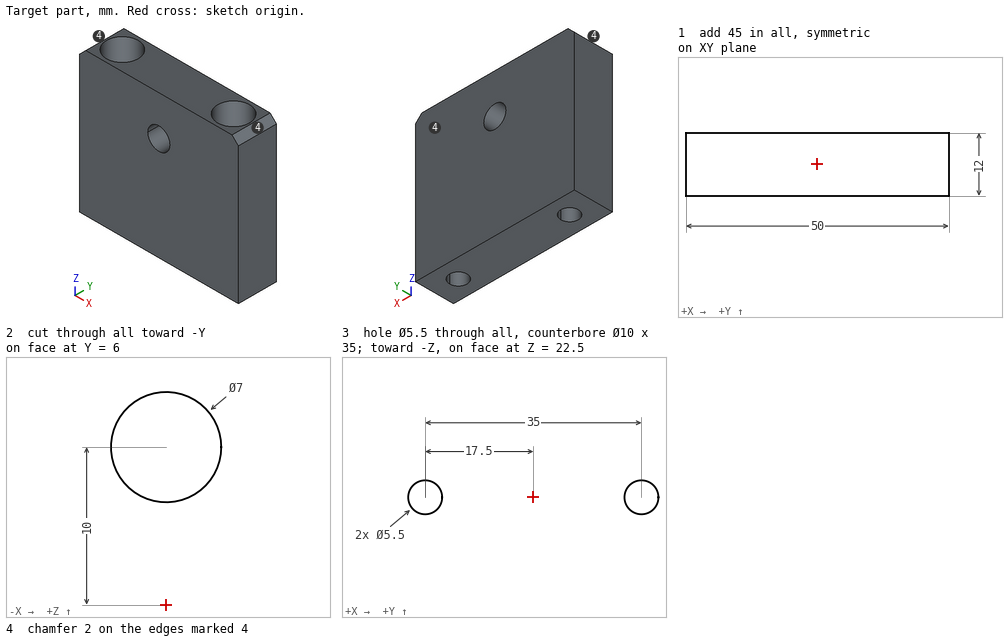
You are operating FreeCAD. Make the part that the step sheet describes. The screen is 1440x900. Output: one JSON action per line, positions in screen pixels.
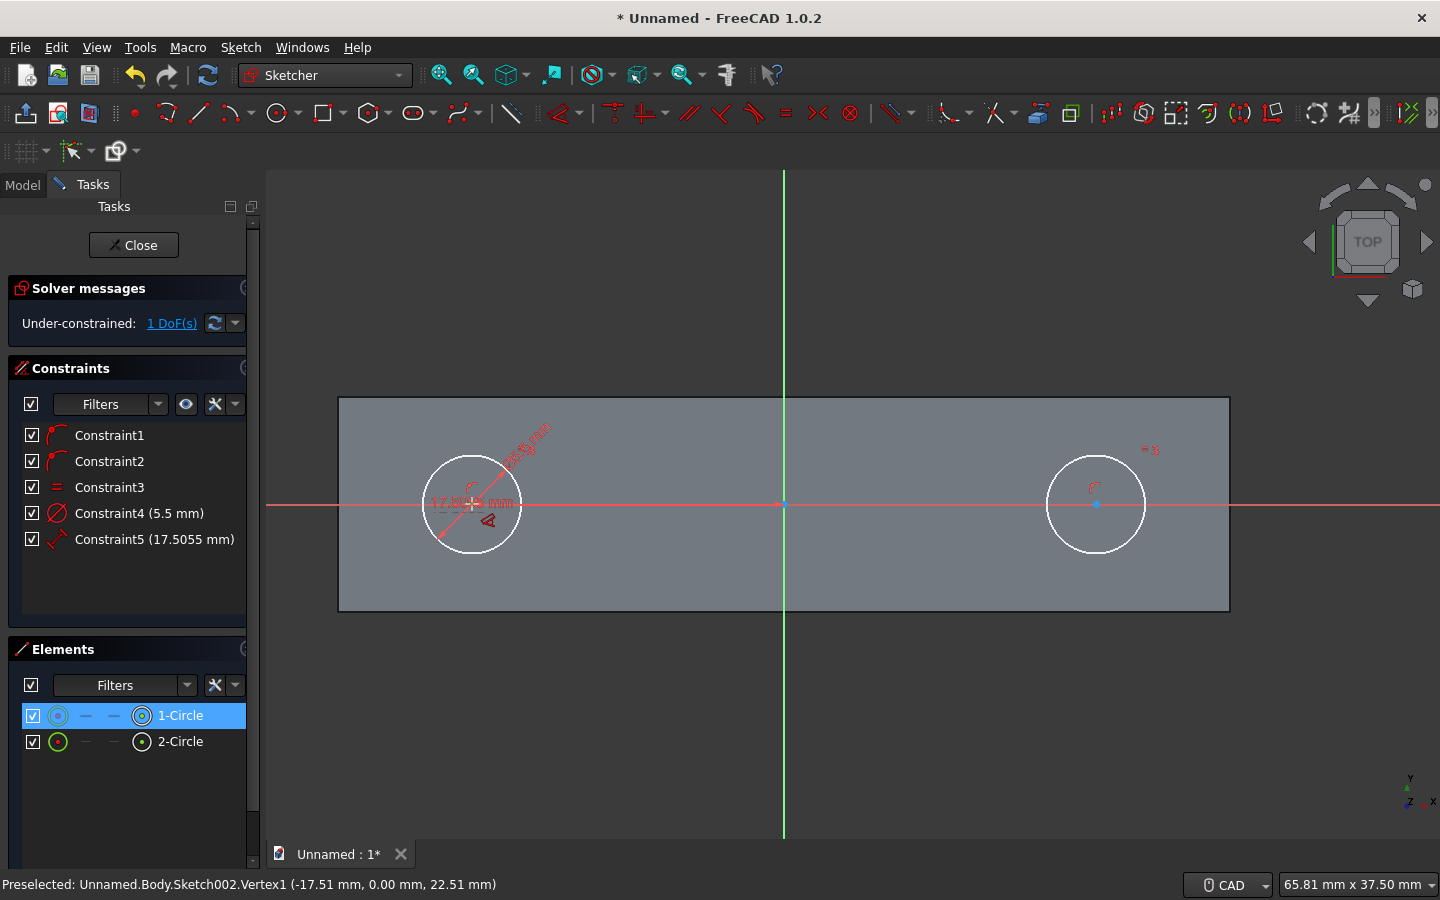
{"action": "left_click", "coordinate": [1096, 504]}
{"action": "left_click", "coordinate": [640, 538]}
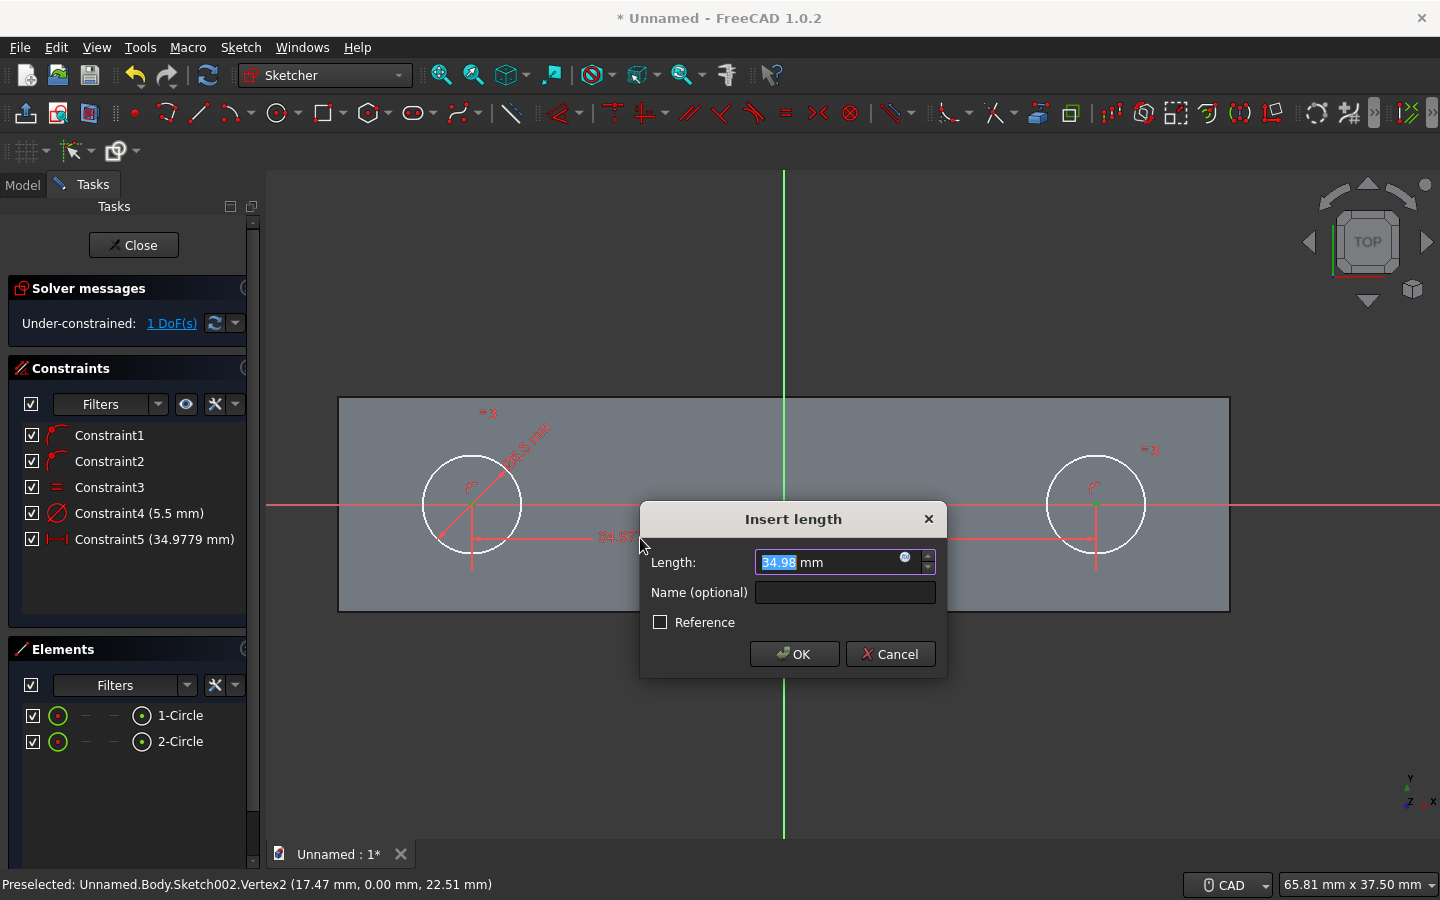
{"action": "type", "text": "35"}
{"action": "key", "text": "Return"}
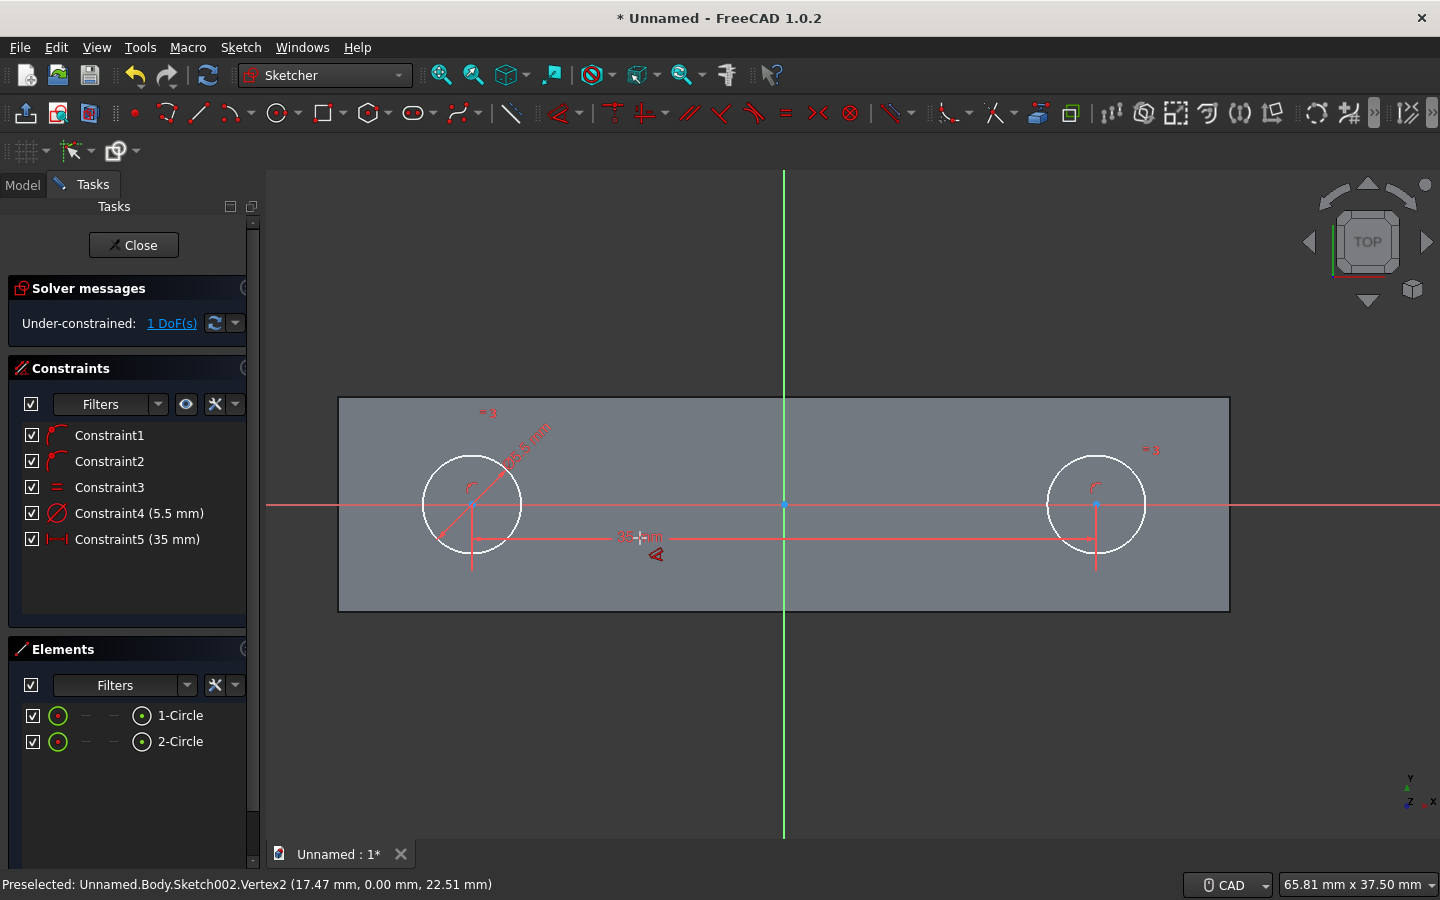
{"action": "left_click", "coordinate": [472, 504]}
{"action": "left_click", "coordinate": [556, 538]}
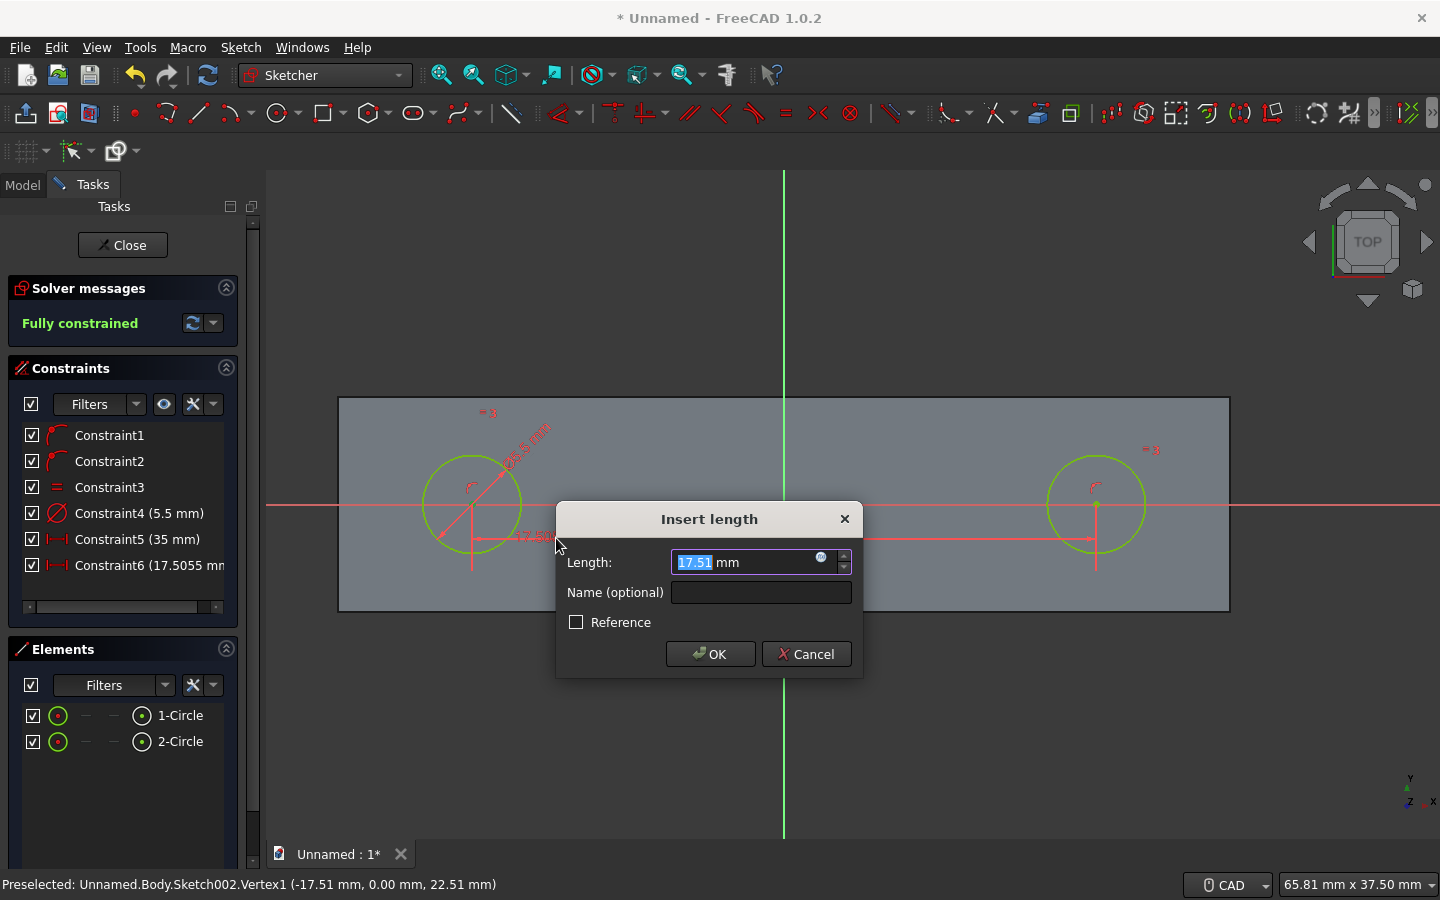
{"action": "type", "text": "17.5"}
{"action": "key", "text": "Return"}
{"action": "key", "text": "Escape"}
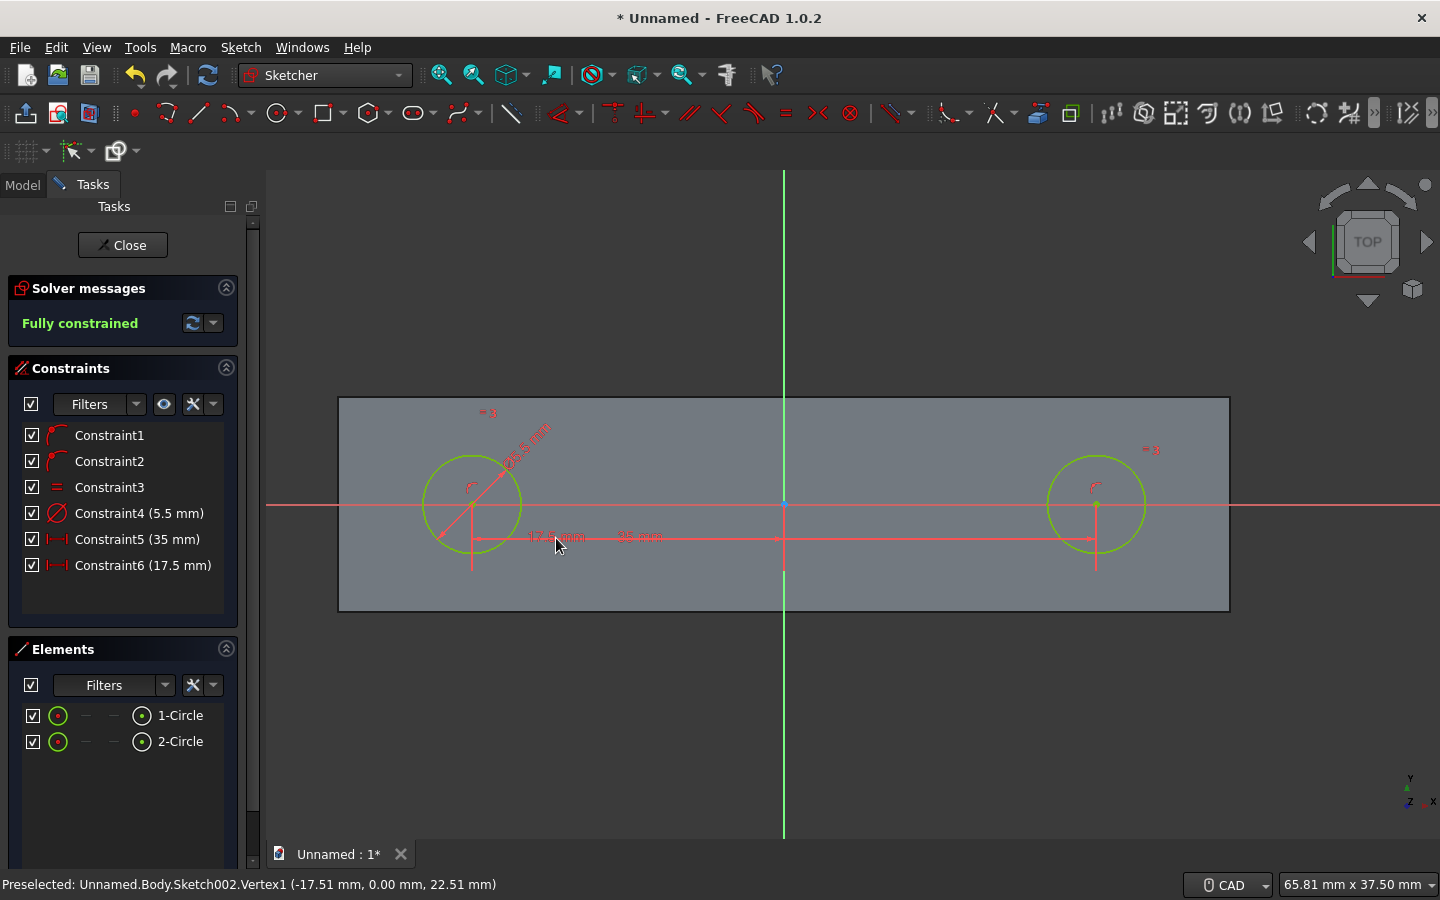
{"action": "left_click", "coordinate": [123, 245]}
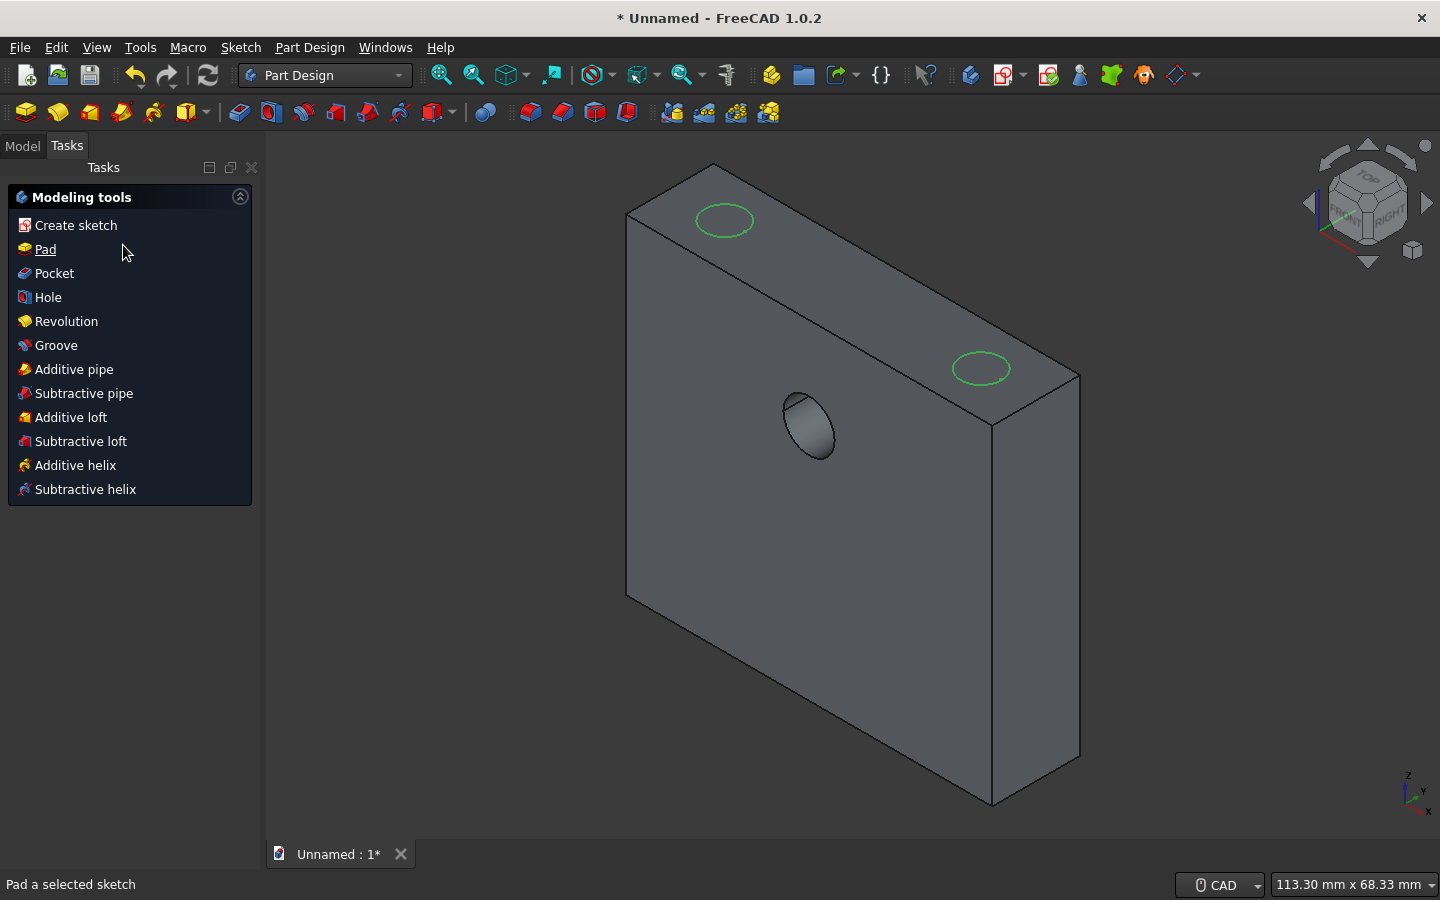
{"action": "left_click", "coordinate": [272, 112]}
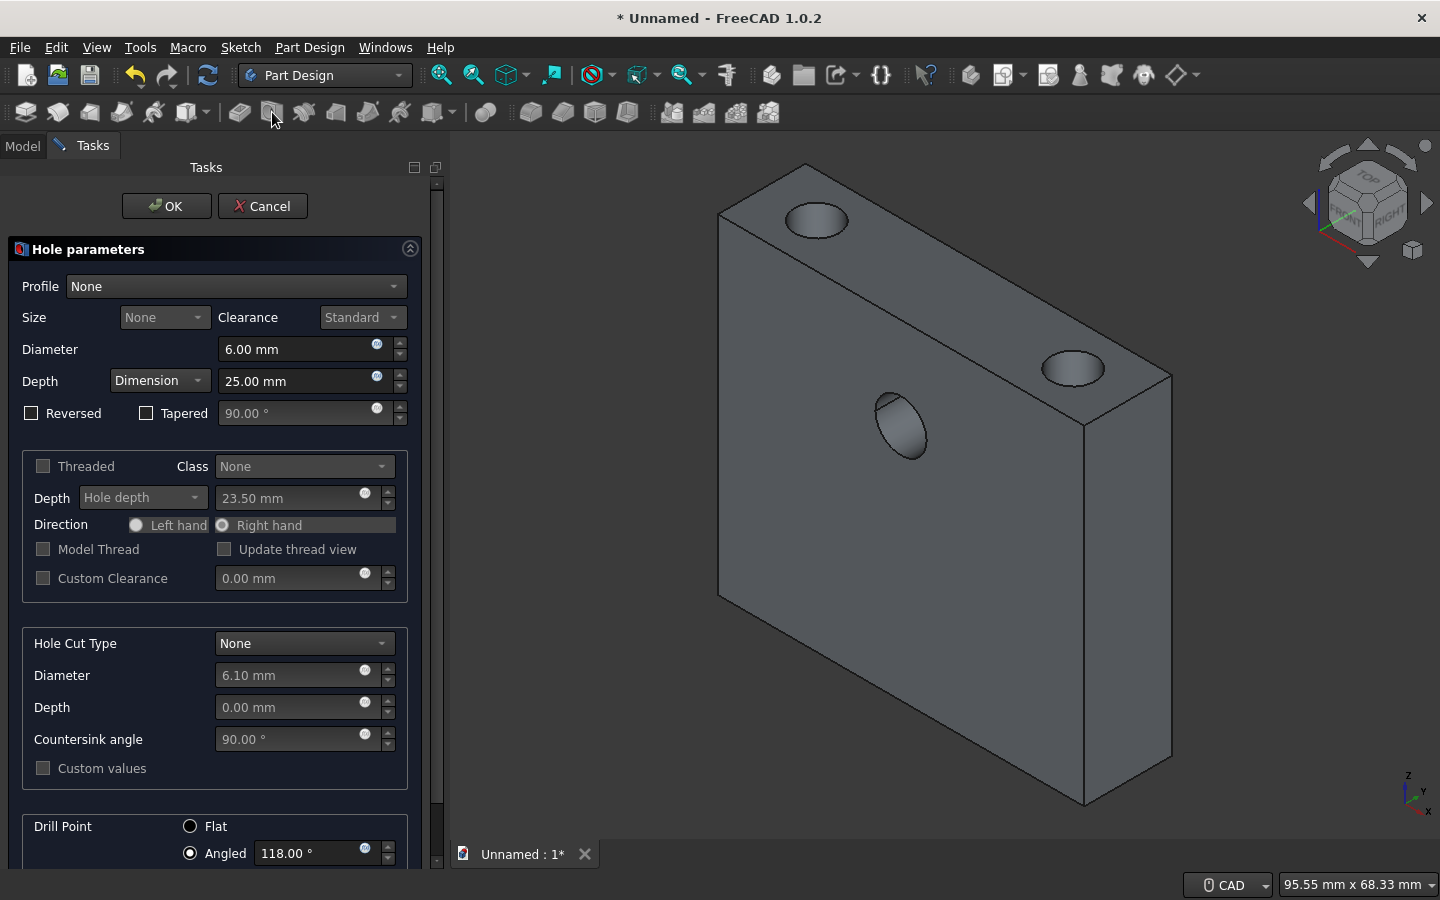
{"action": "triple_click", "coordinate": [305, 349]}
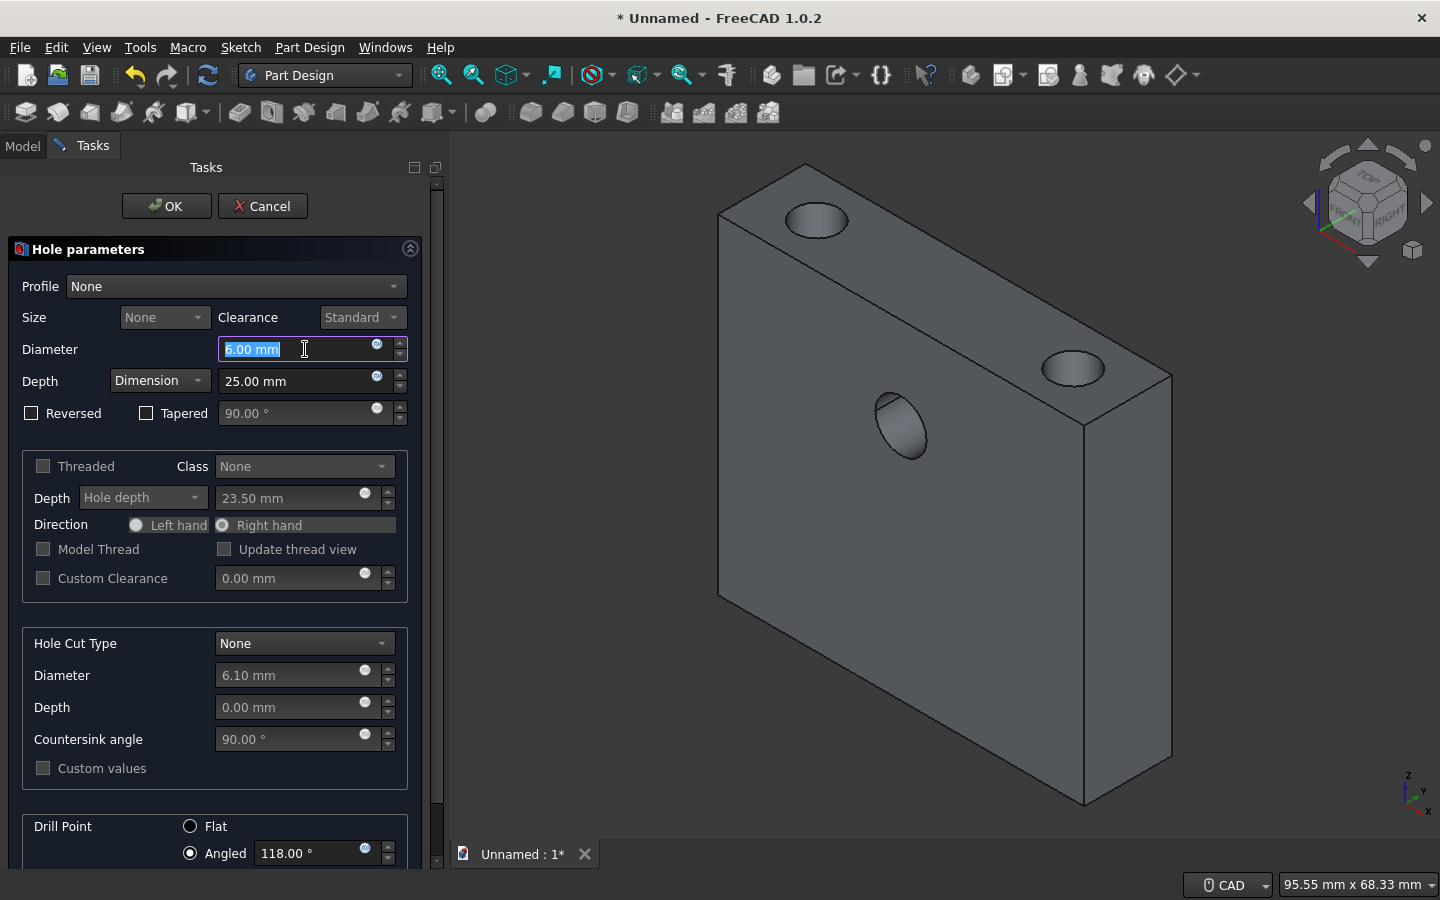
{"action": "type", "text": "5.5"}
{"action": "key", "text": "Tab"}